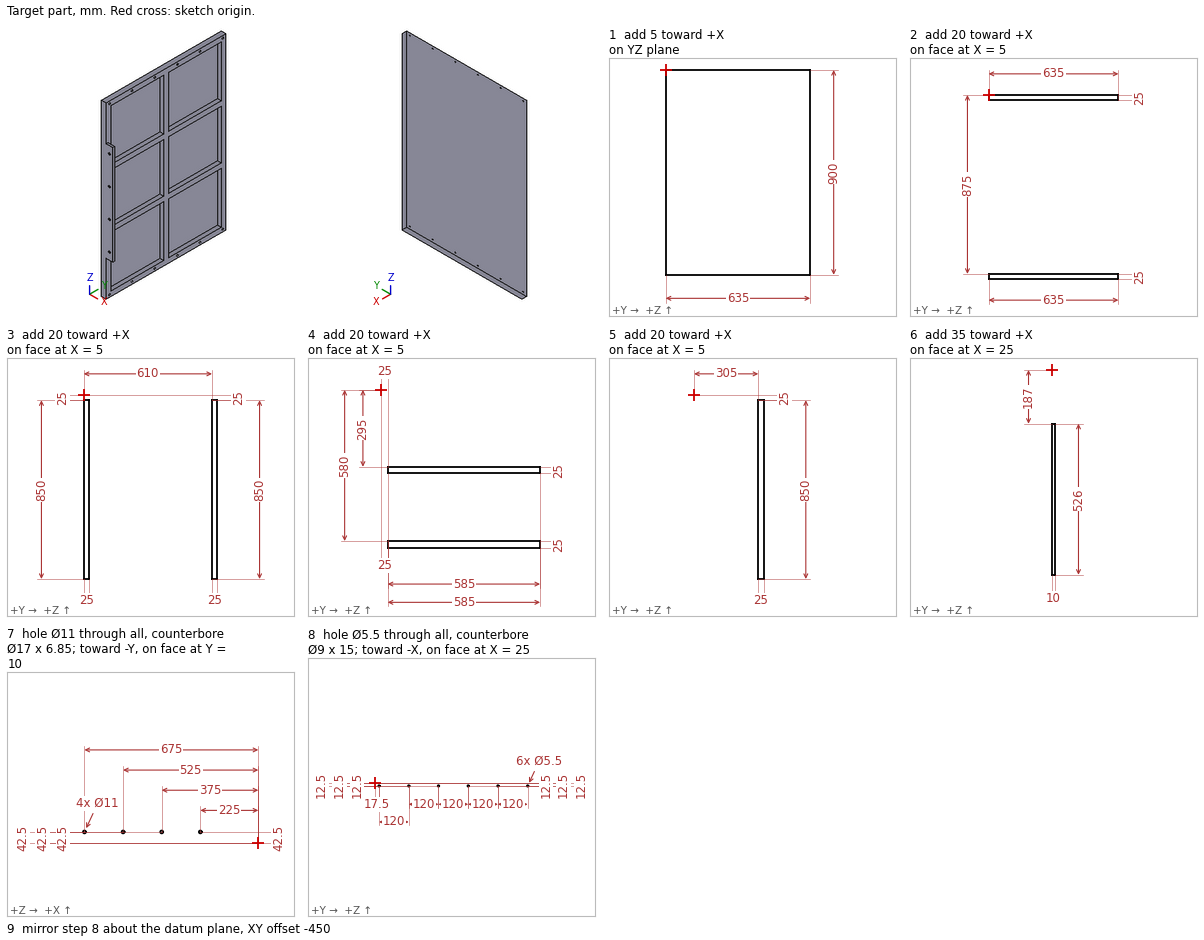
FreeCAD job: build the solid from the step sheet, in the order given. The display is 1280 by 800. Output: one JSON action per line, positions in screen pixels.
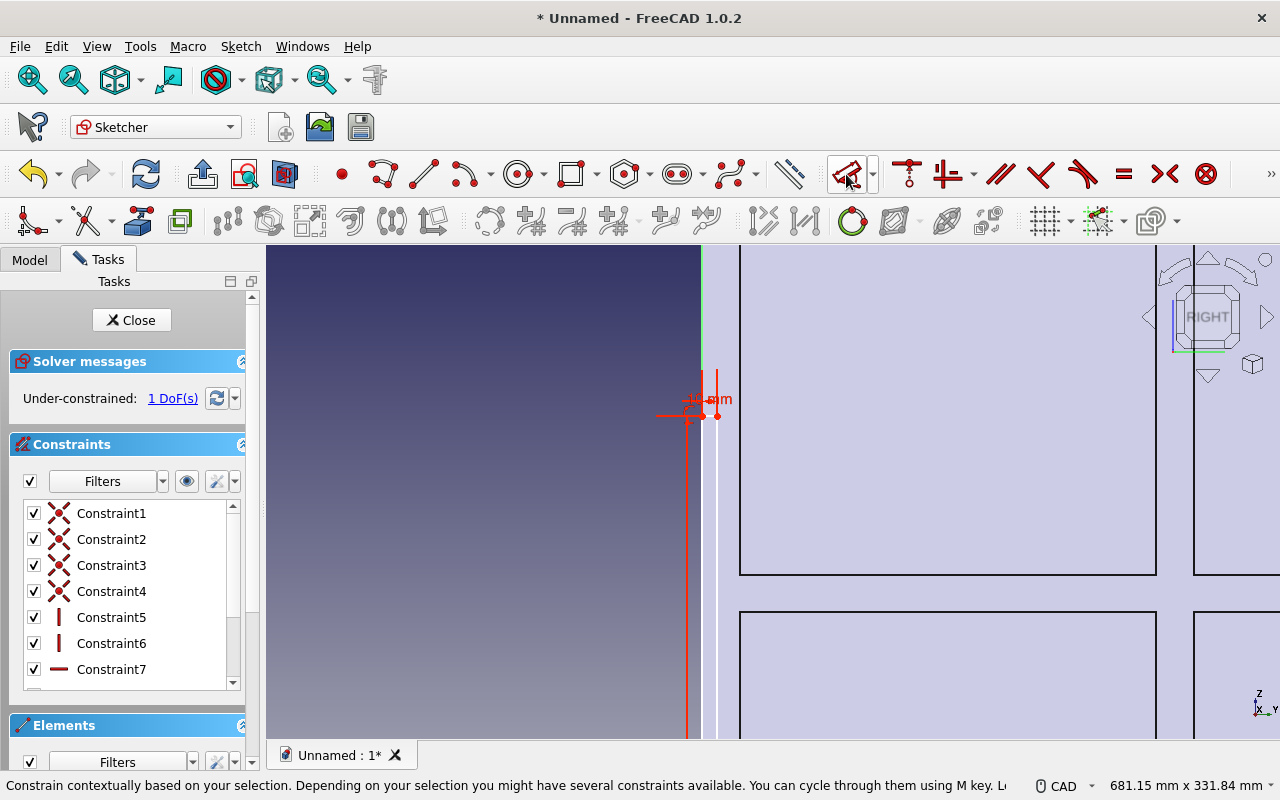
{"action": "left_click", "coordinate": [702, 416]}
{"action": "left_click", "coordinate": [668, 345]}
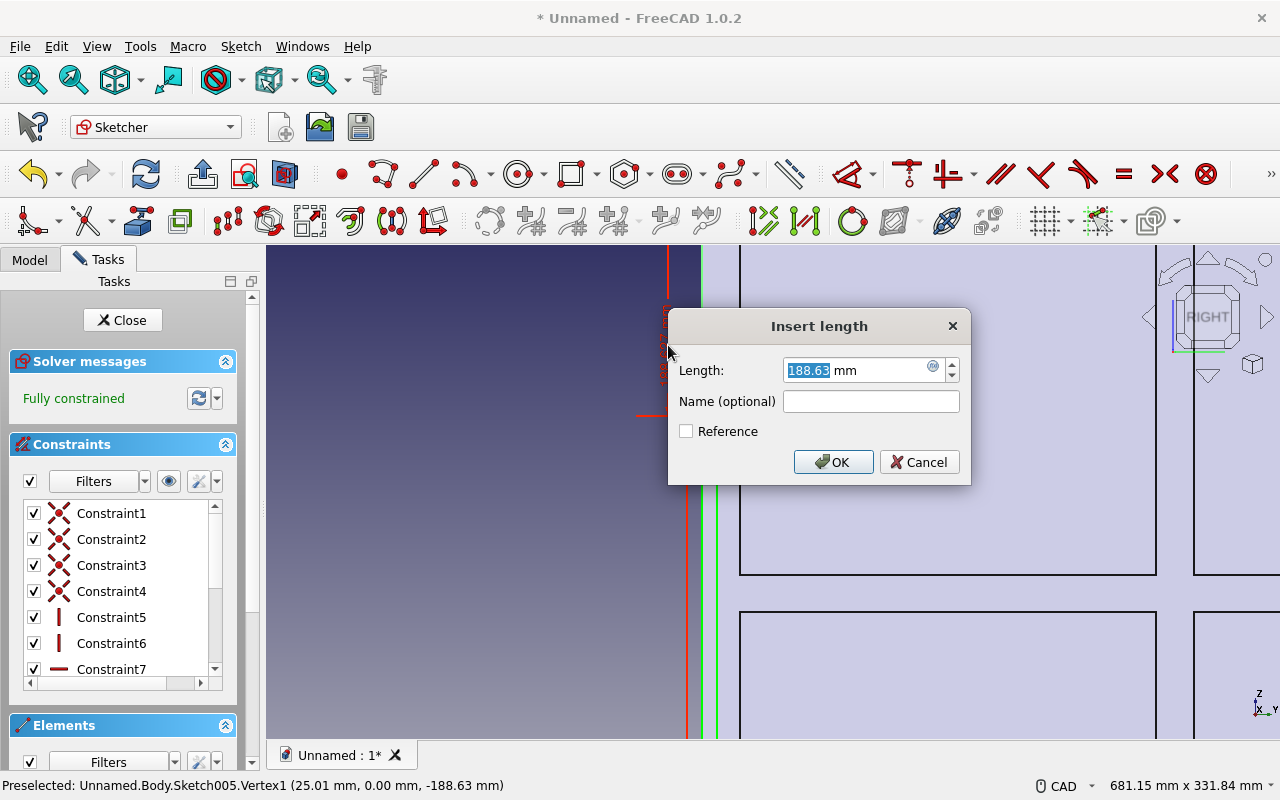
{"action": "type", "text": "187"}
{"action": "key", "text": "Return"}
{"action": "key", "text": "Escape"}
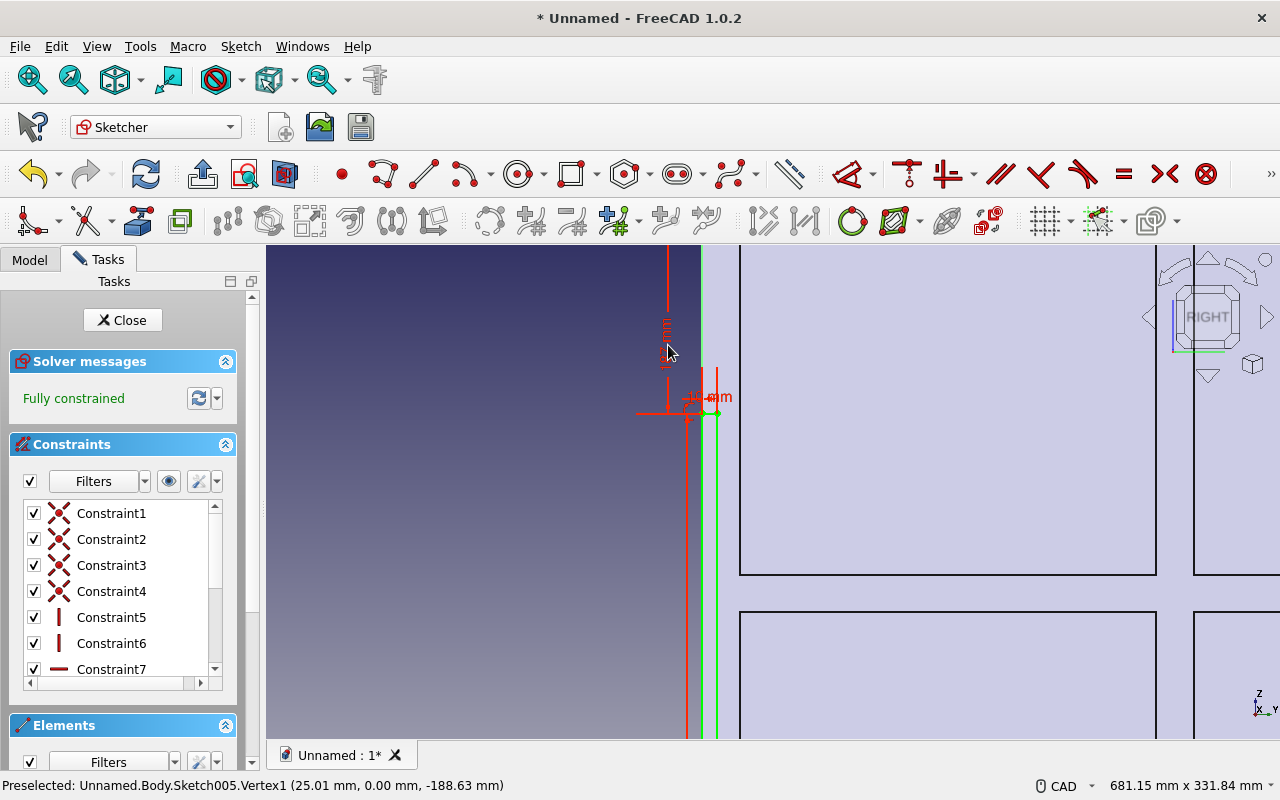
{"action": "left_click", "coordinate": [123, 320]}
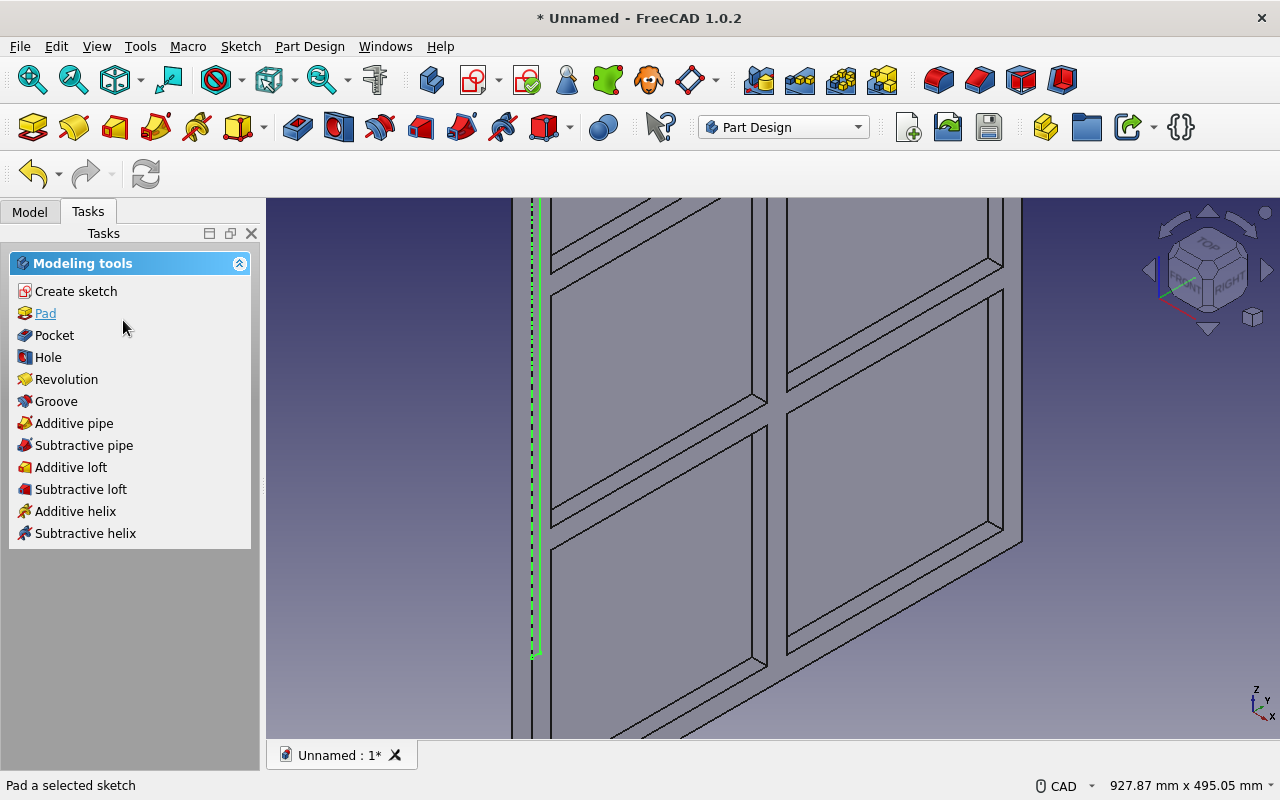
{"action": "left_click", "coordinate": [33, 128]}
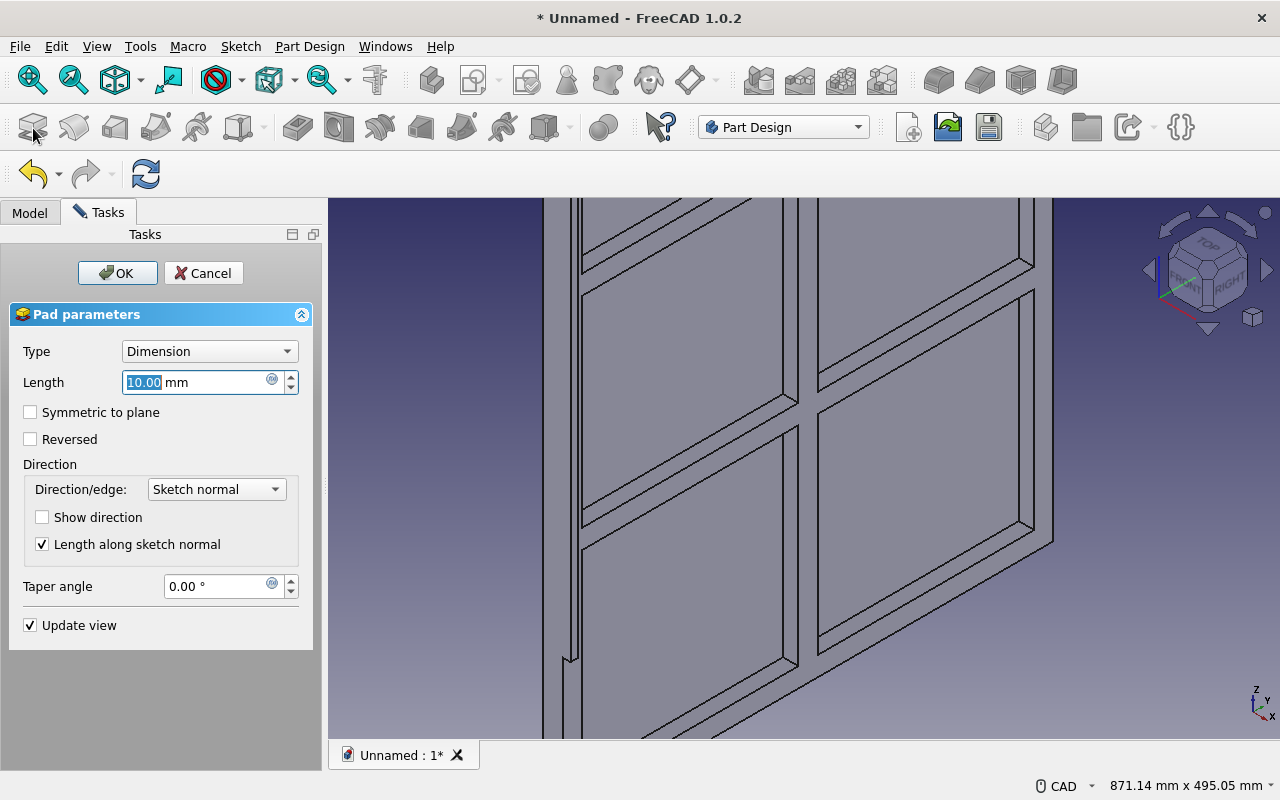
{"action": "type", "text": "35"}
{"action": "key", "text": "Tab"}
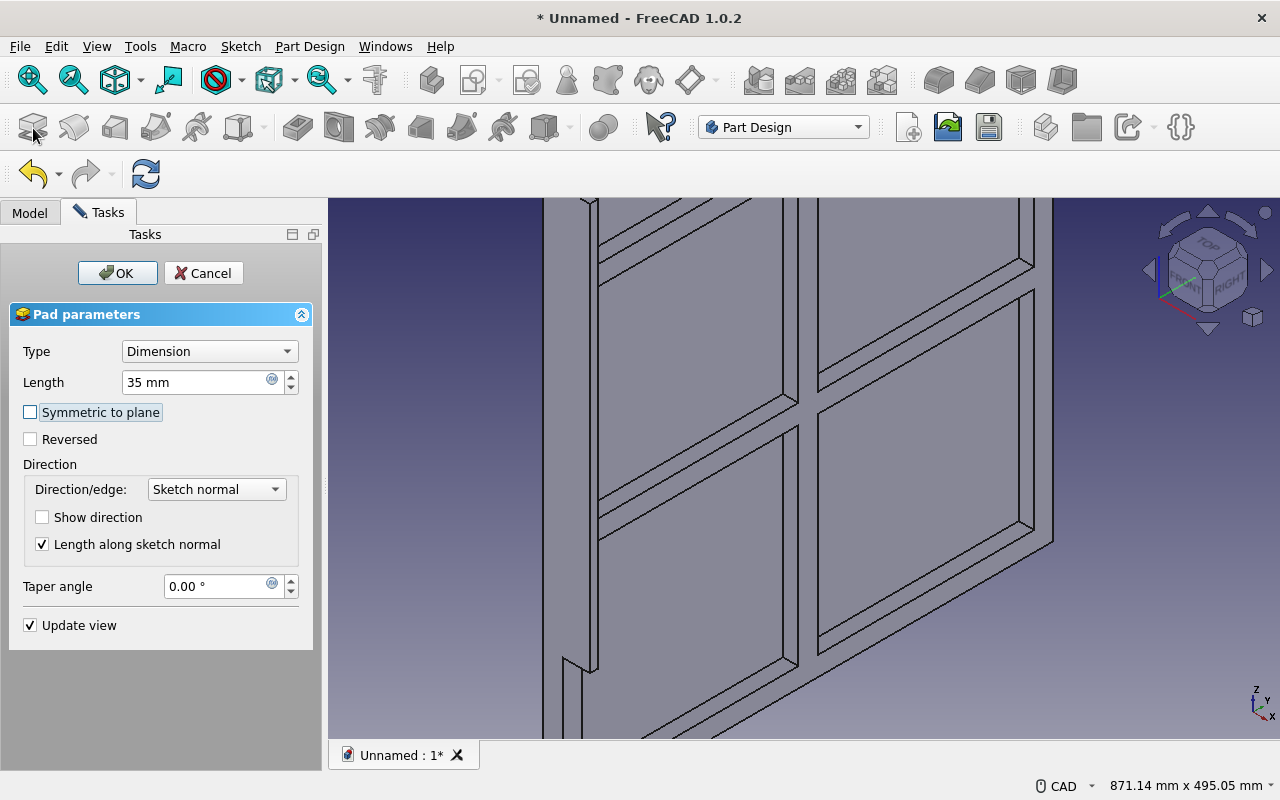
{"action": "left_click", "coordinate": [118, 273]}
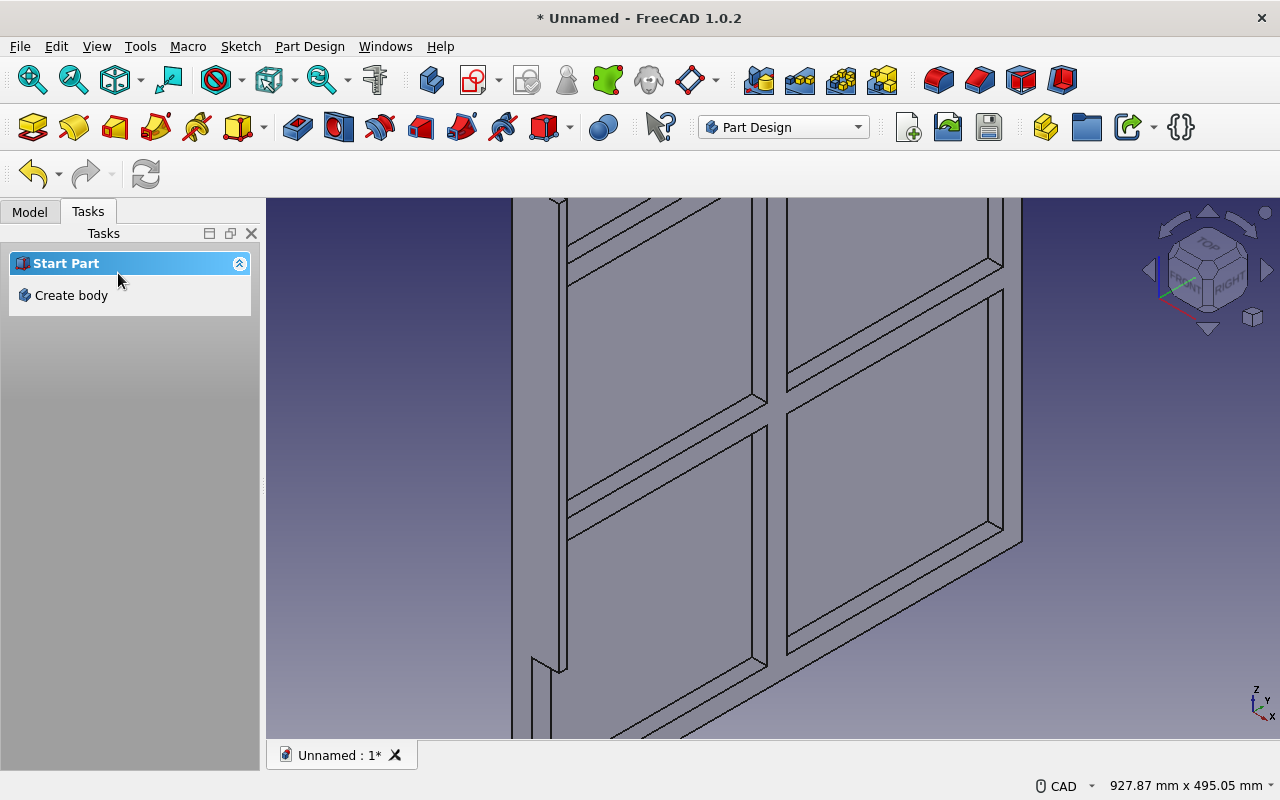
{"action": "left_click", "coordinate": [33, 80]}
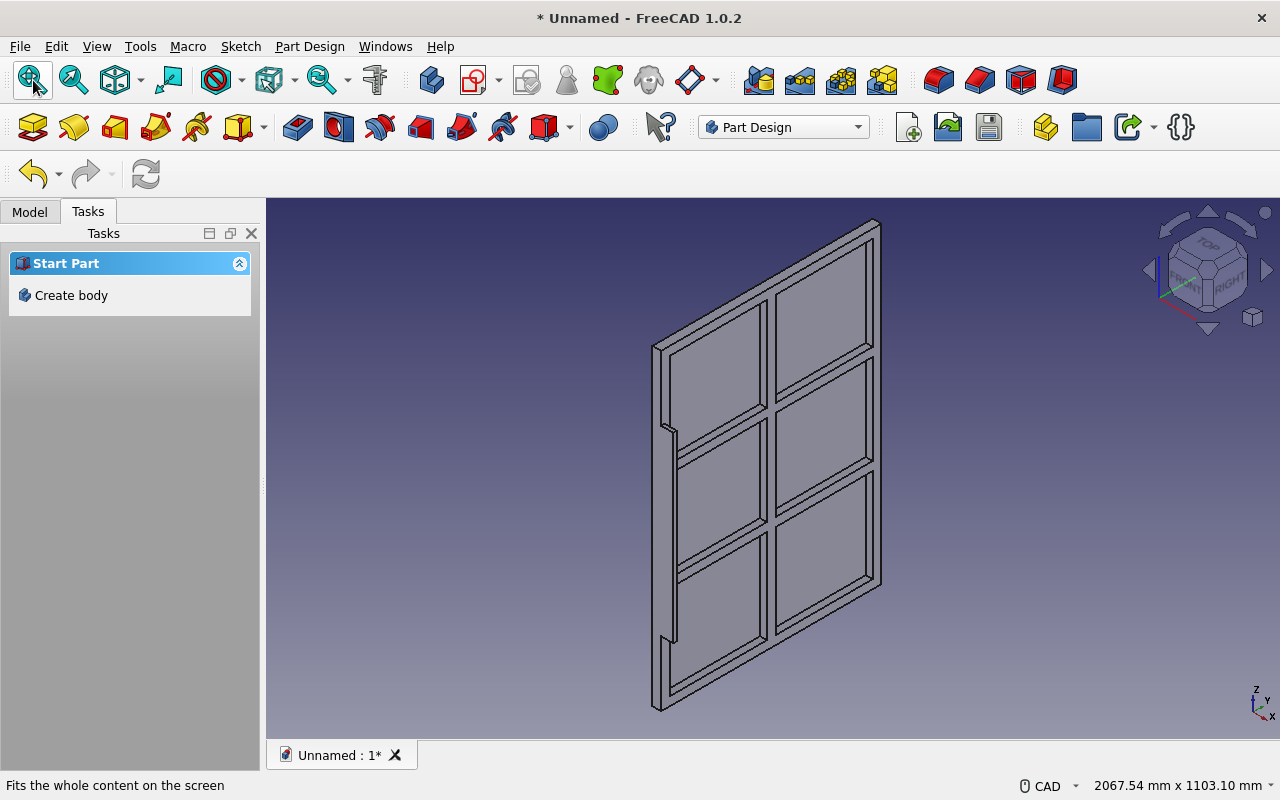
{"action": "key", "text": "4"}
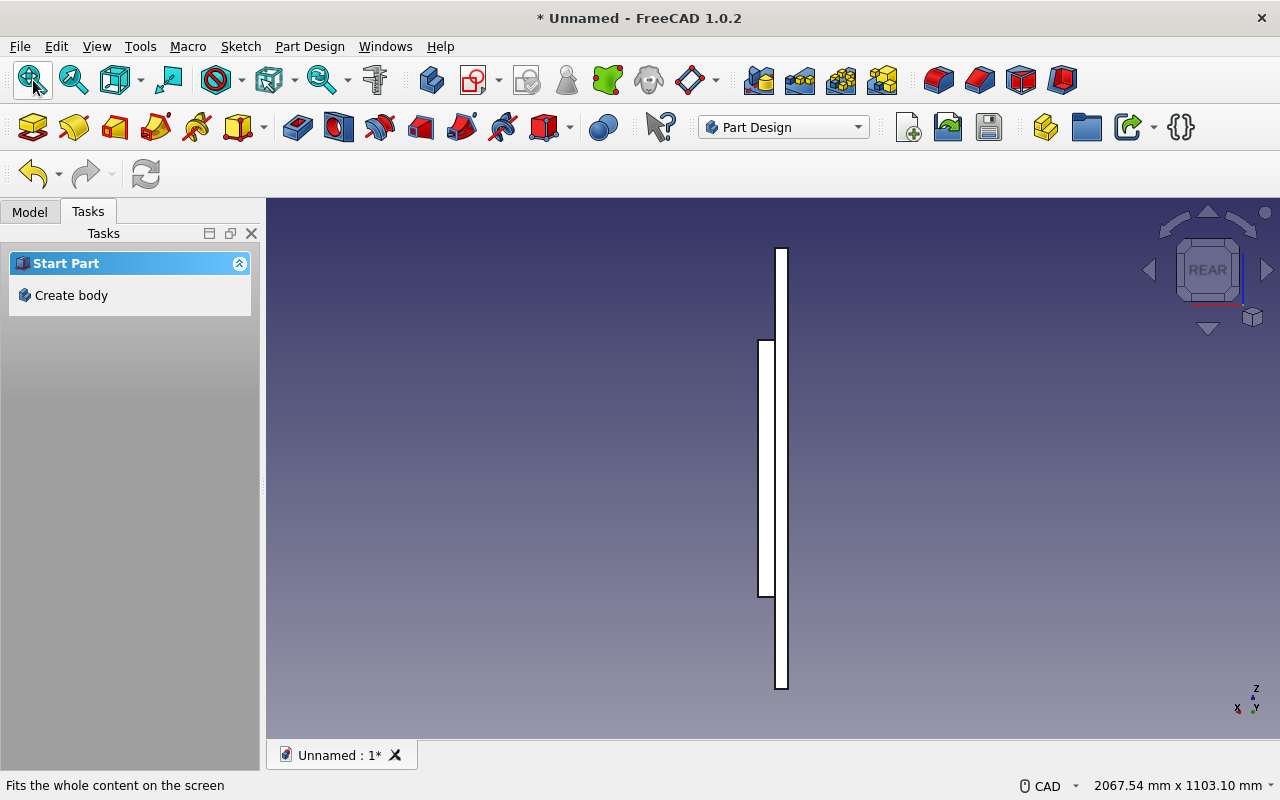
{"action": "left_click", "coordinate": [767, 541]}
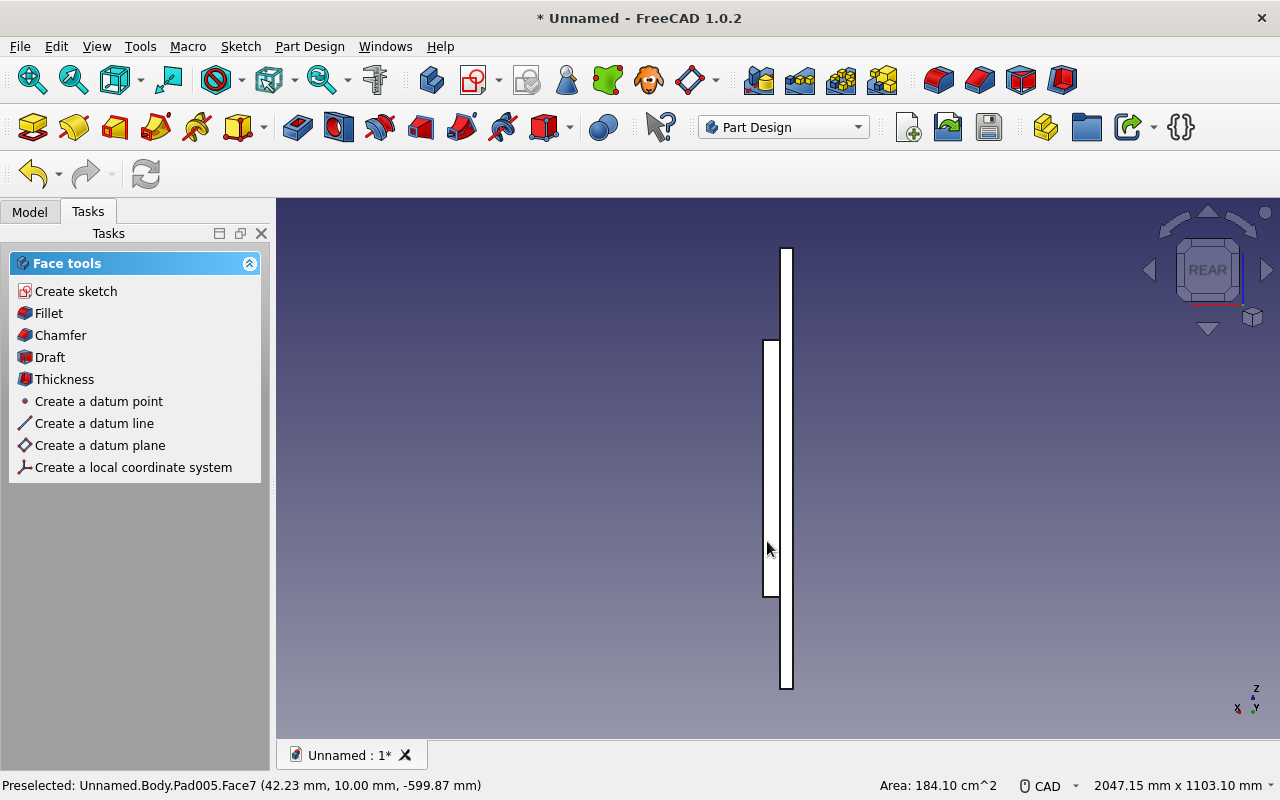
{"action": "left_click", "coordinate": [472, 80]}